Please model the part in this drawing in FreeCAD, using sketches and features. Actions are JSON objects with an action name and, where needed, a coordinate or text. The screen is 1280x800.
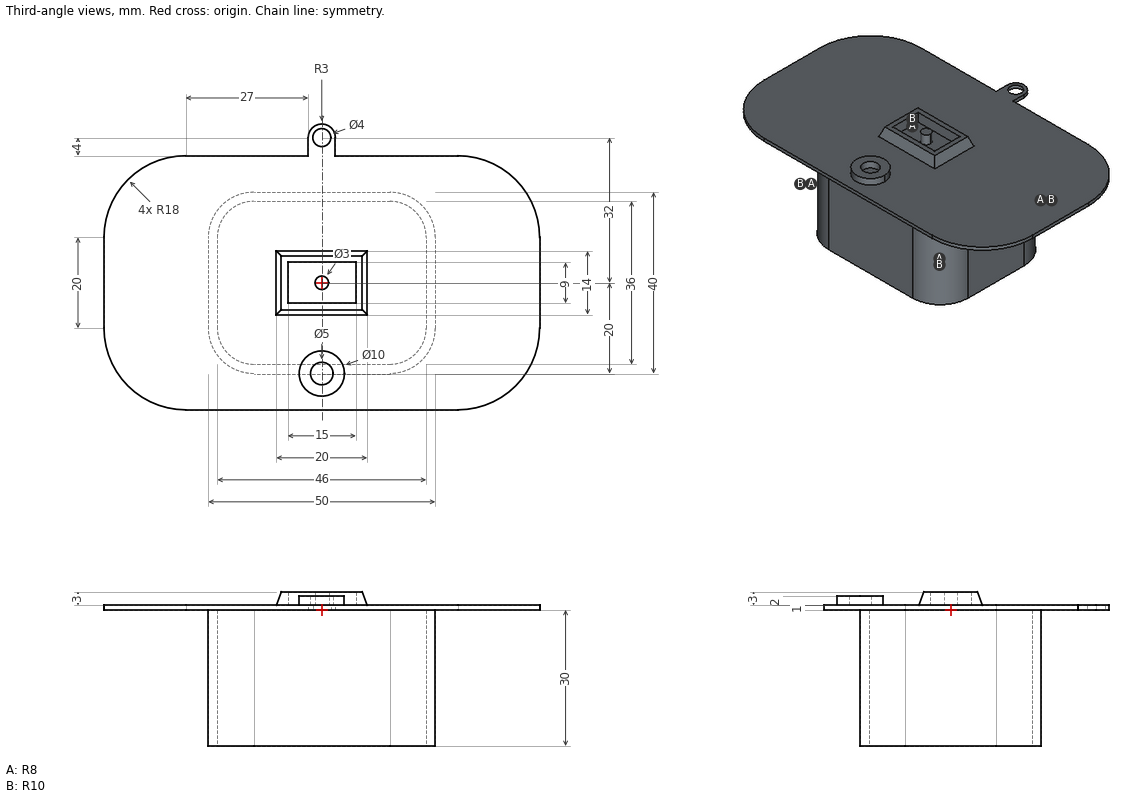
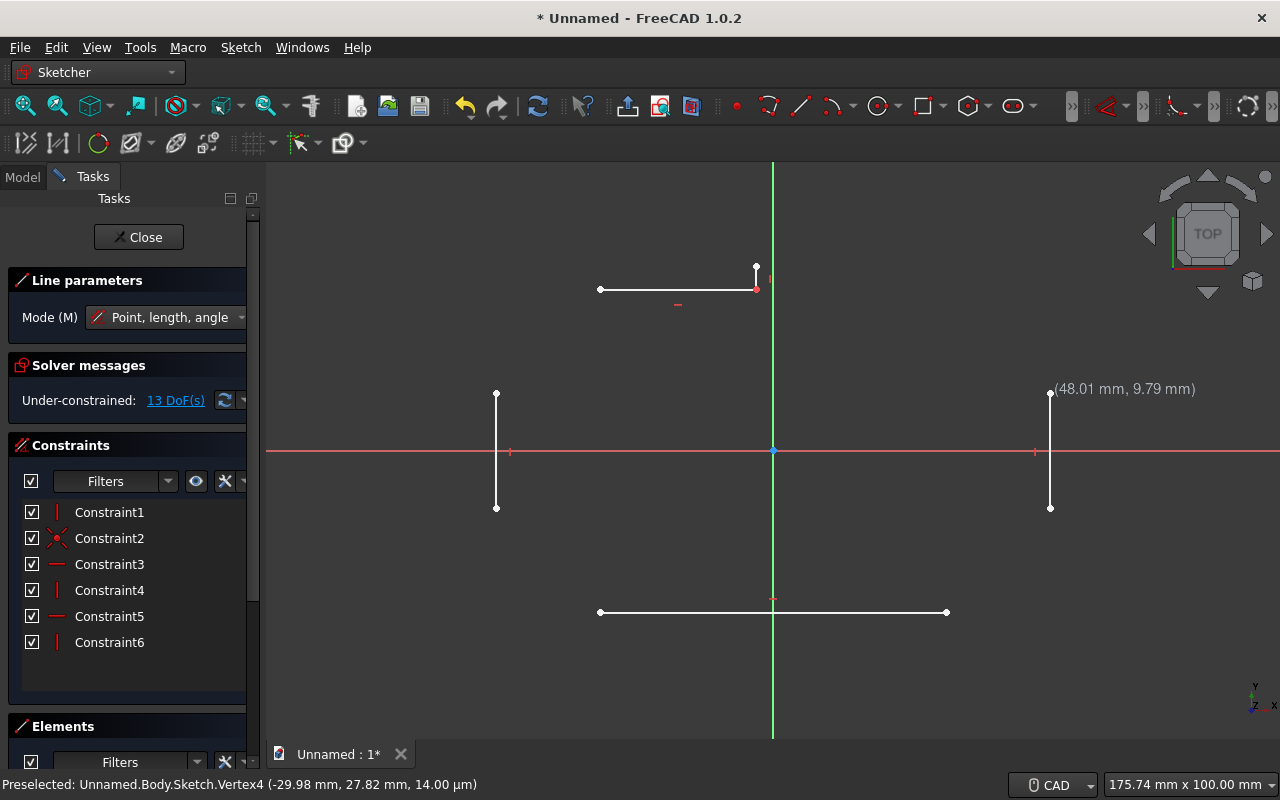
{"action": "left_click", "coordinate": [770, 106]}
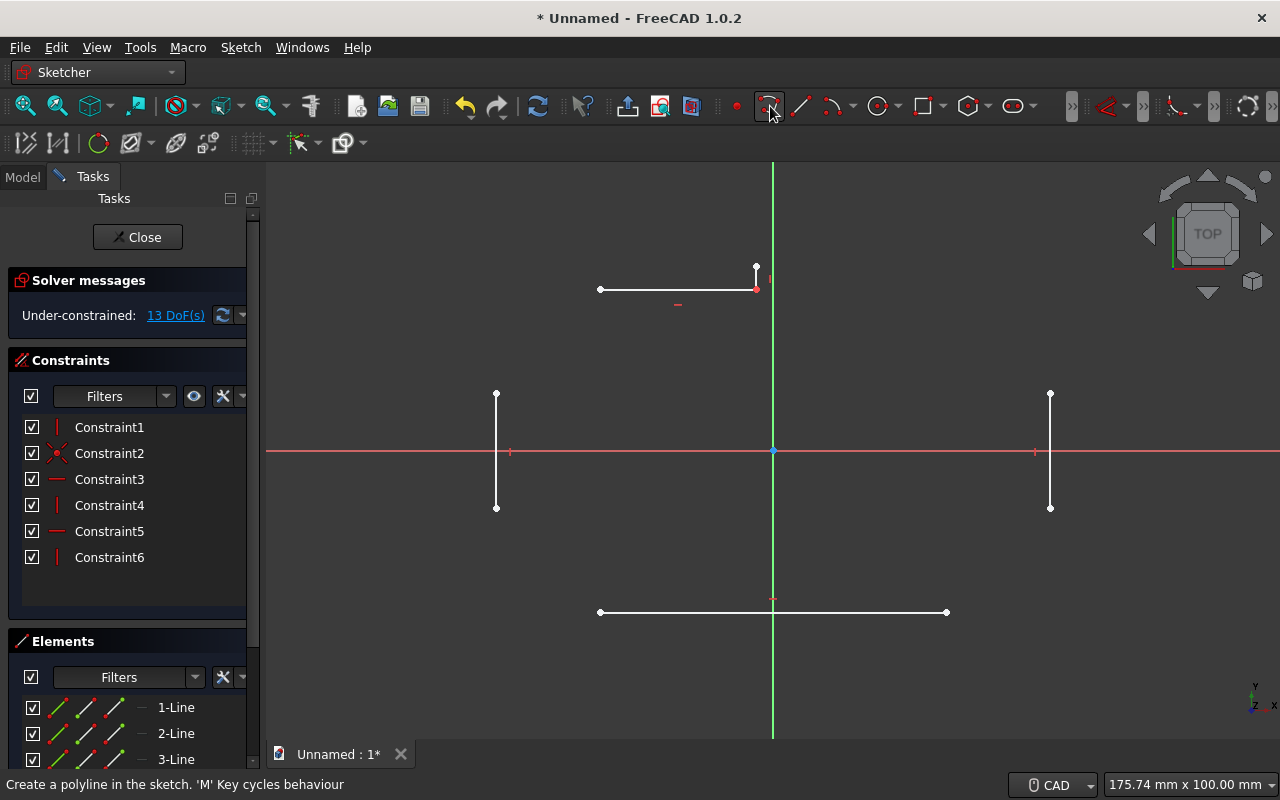
{"action": "left_click", "coordinate": [946, 289]}
{"action": "left_click", "coordinate": [790, 289]}
{"action": "left_click", "coordinate": [790, 266]}
{"action": "right_click", "coordinate": [790, 266]}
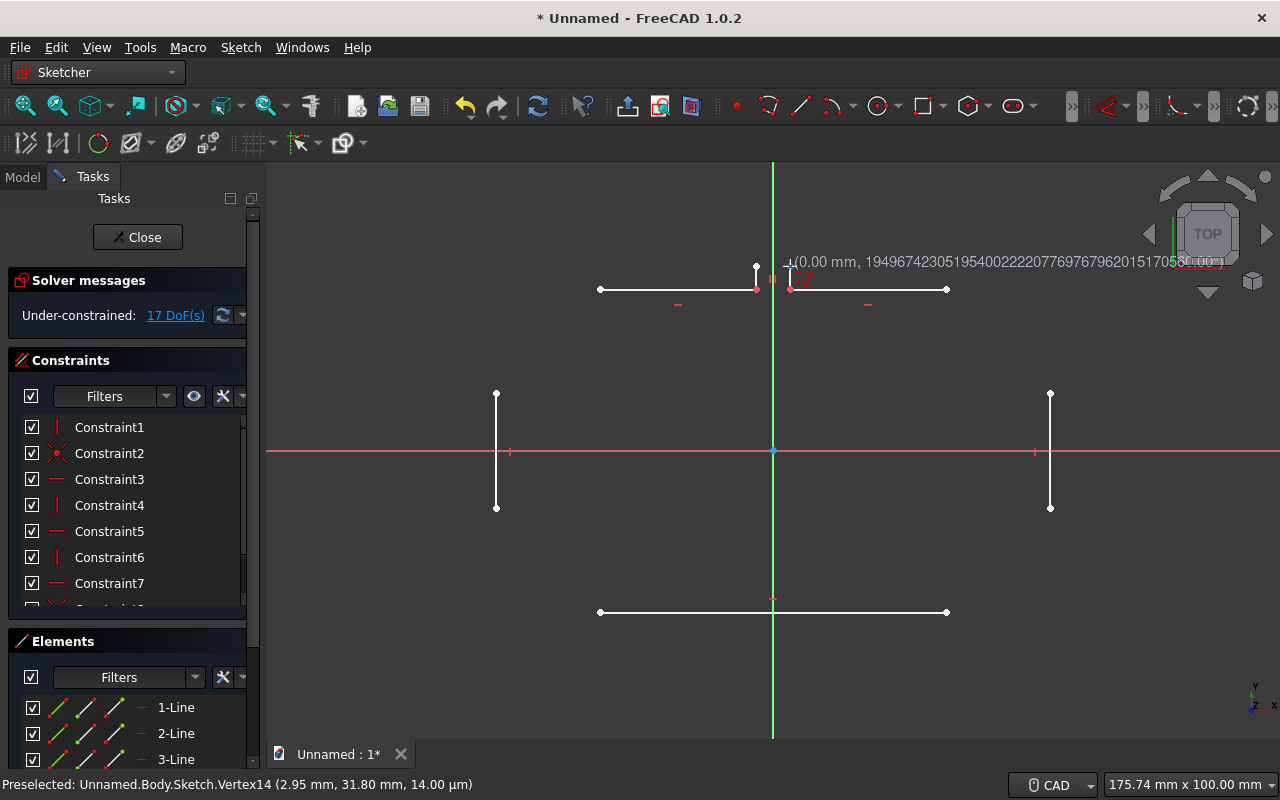
{"action": "key", "text": "g 3 a"}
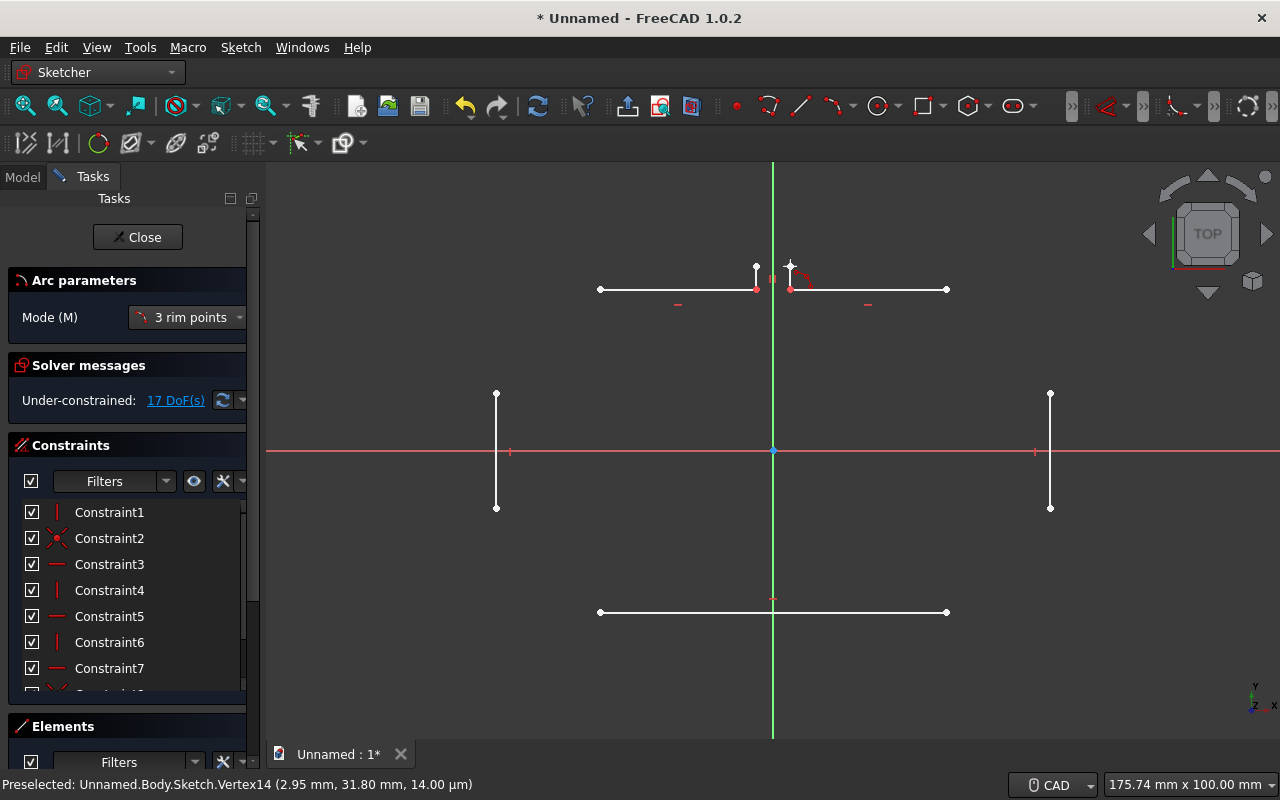
{"action": "left_click", "coordinate": [600, 290]}
{"action": "left_click", "coordinate": [496, 394]}
{"action": "left_click", "coordinate": [526, 319]}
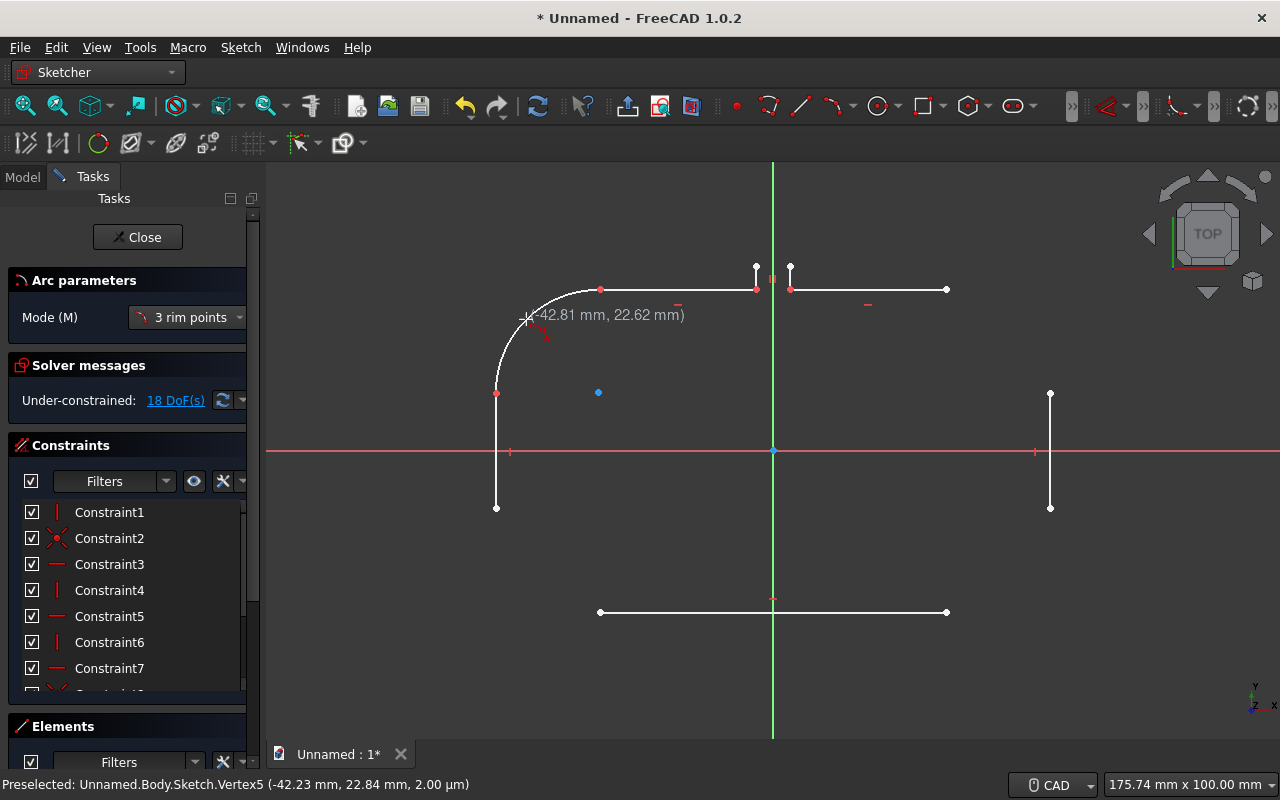
{"action": "left_click", "coordinate": [496, 509]}
{"action": "left_click", "coordinate": [600, 613]}
{"action": "left_click", "coordinate": [526, 582]}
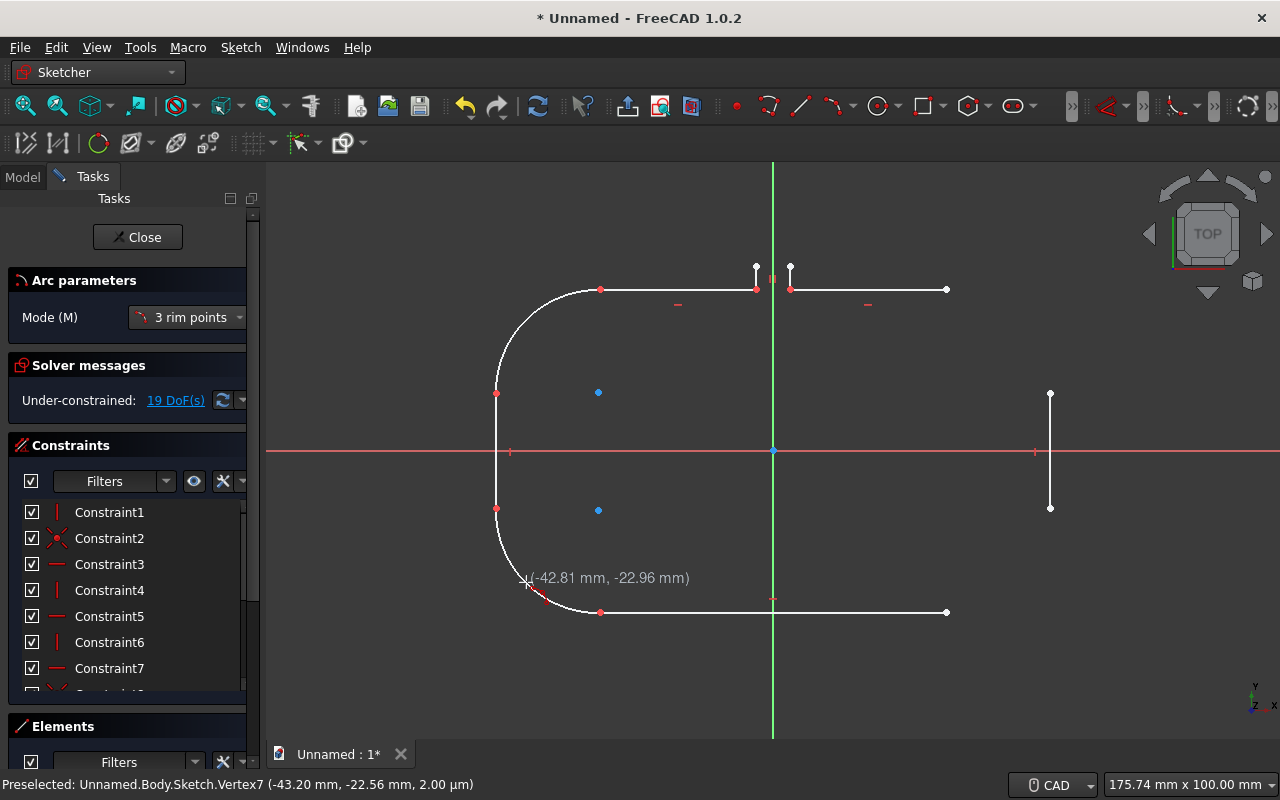
{"action": "left_click", "coordinate": [946, 613]}
{"action": "left_click", "coordinate": [1050, 509]}
{"action": "left_click", "coordinate": [1020, 582]}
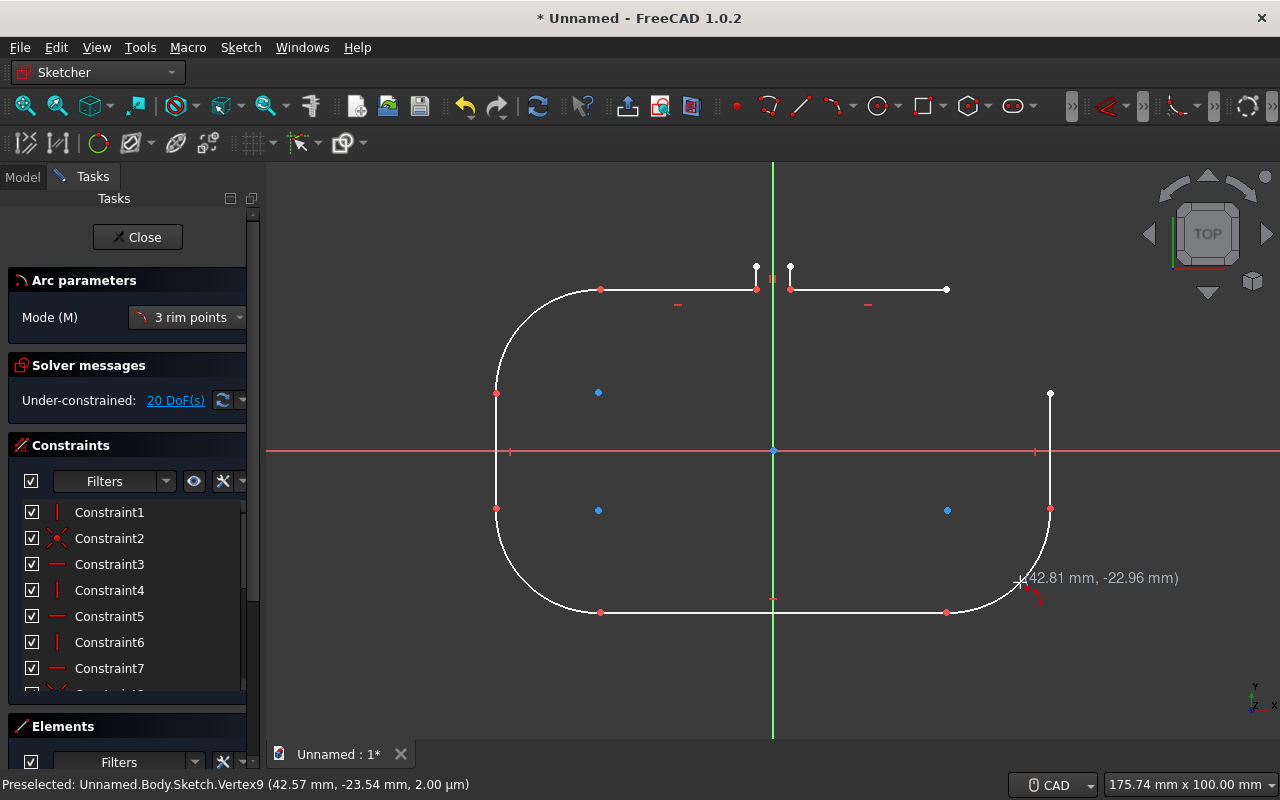
{"action": "left_click", "coordinate": [1050, 394]}
{"action": "left_click", "coordinate": [946, 290]}
{"action": "left_click", "coordinate": [1020, 319]}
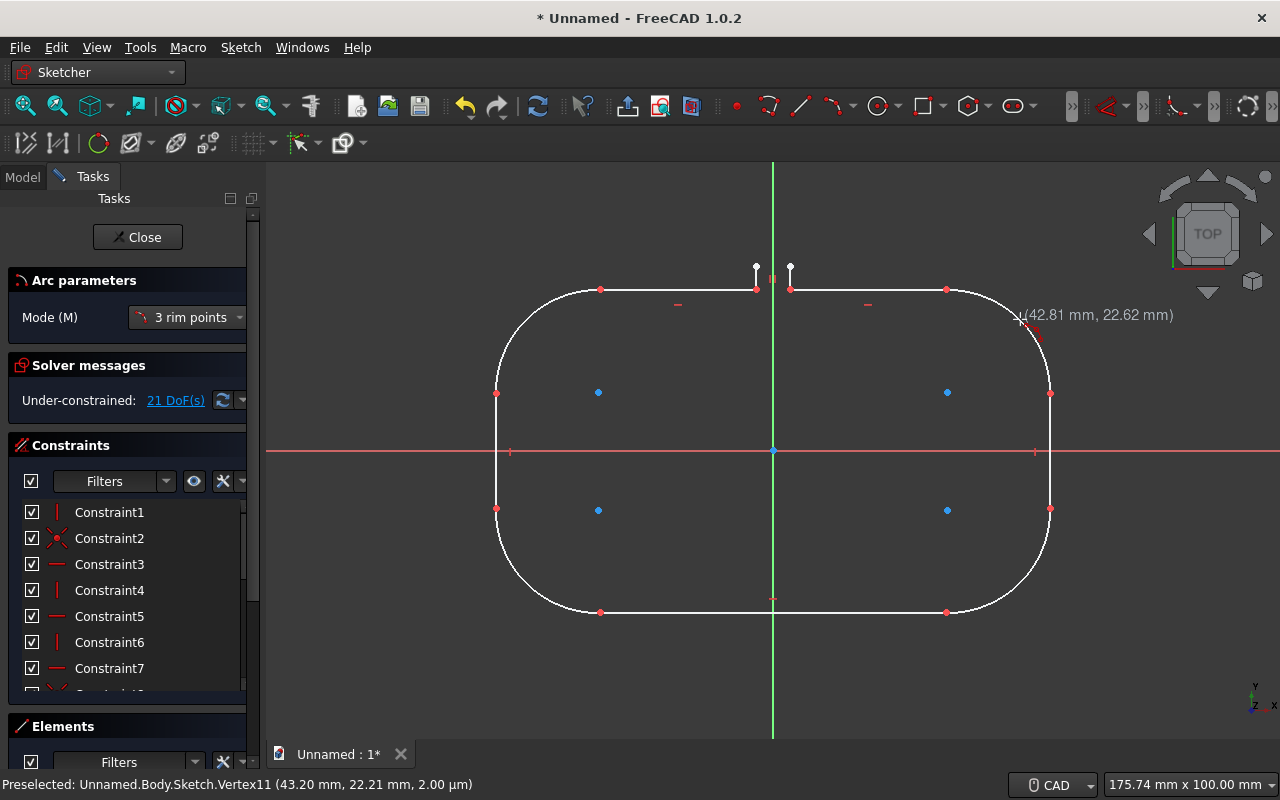
{"action": "scroll", "coordinate": [790, 266], "scroll_direction": "up", "scroll_amount": 2}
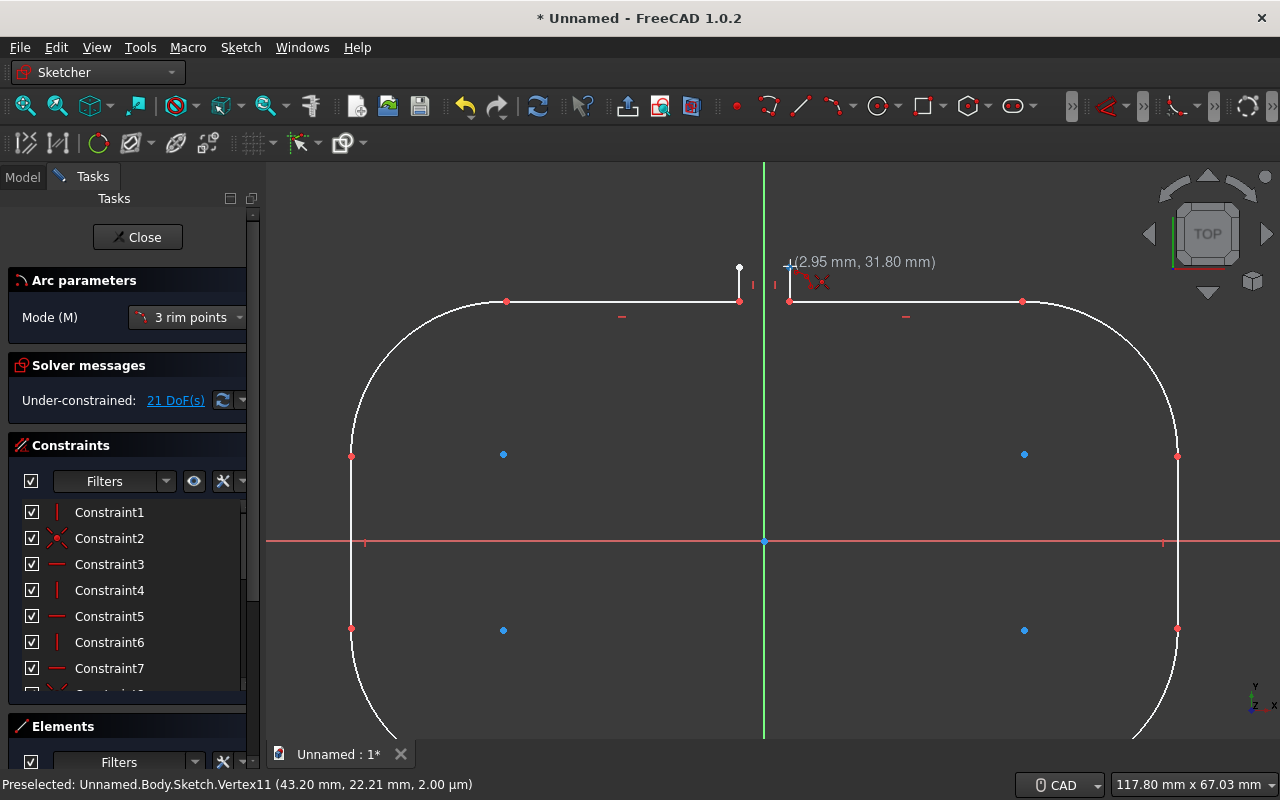
{"action": "left_click", "coordinate": [790, 267]}
{"action": "left_click", "coordinate": [739, 267]}
{"action": "left_click", "coordinate": [780, 245]}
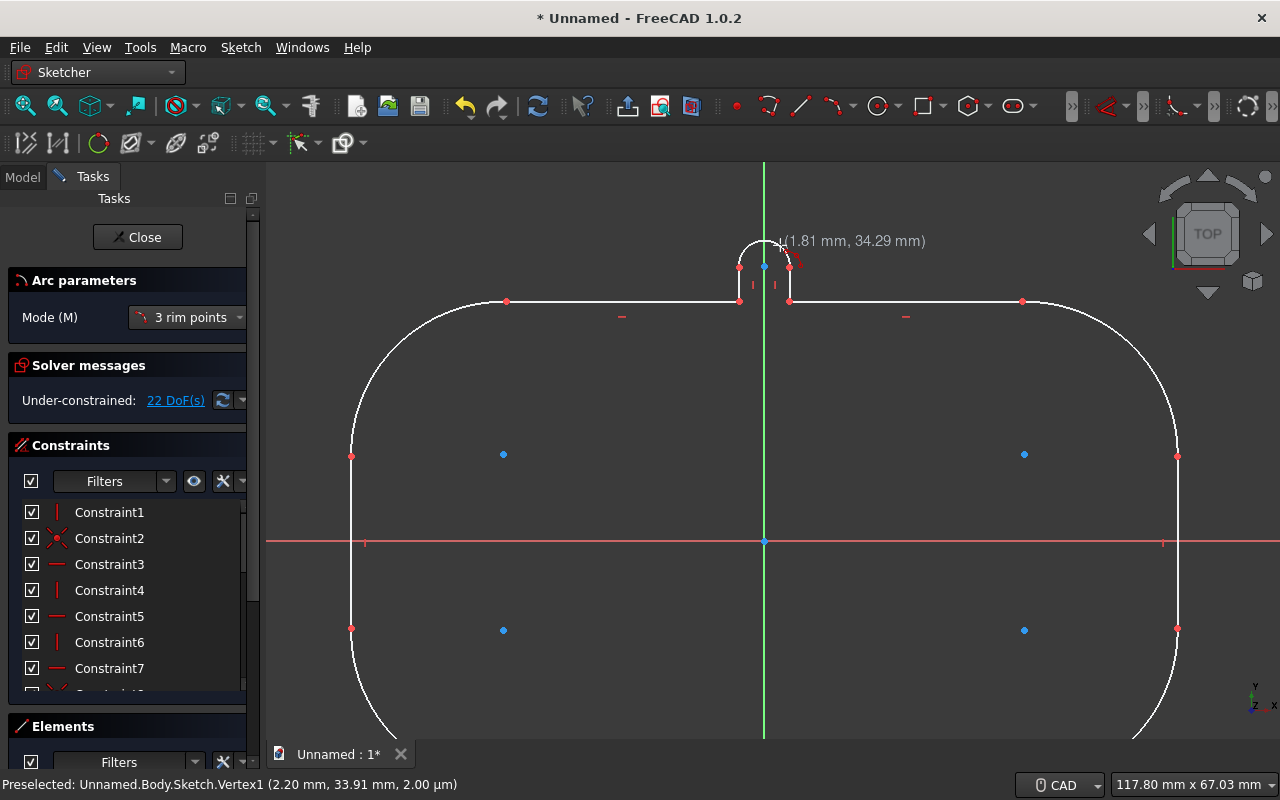
{"action": "left_click", "coordinate": [878, 106]}